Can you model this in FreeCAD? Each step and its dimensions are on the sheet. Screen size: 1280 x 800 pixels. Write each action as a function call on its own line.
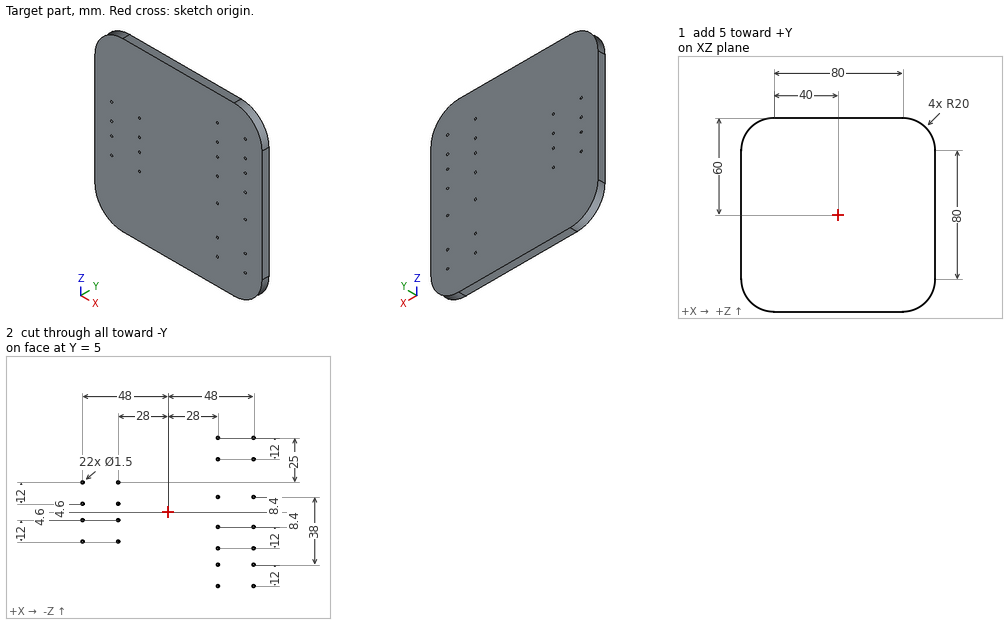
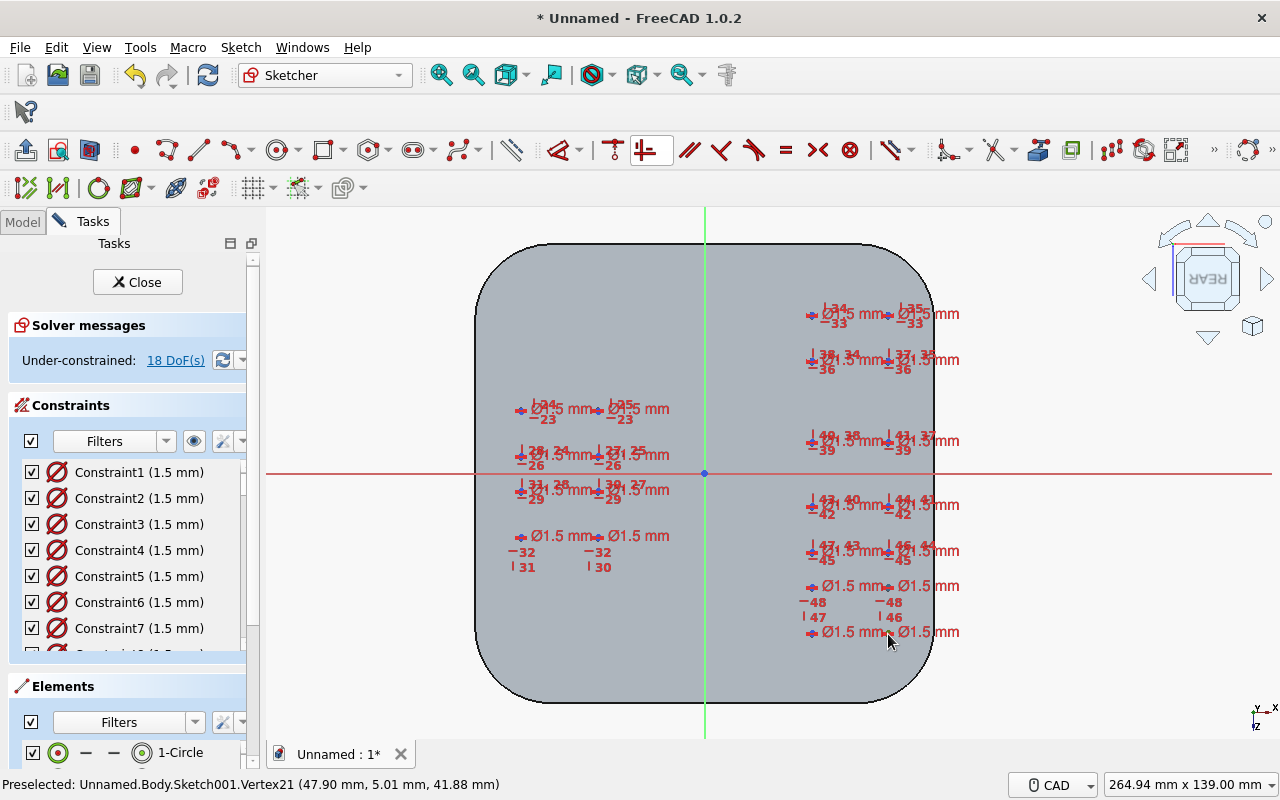
click(668, 150)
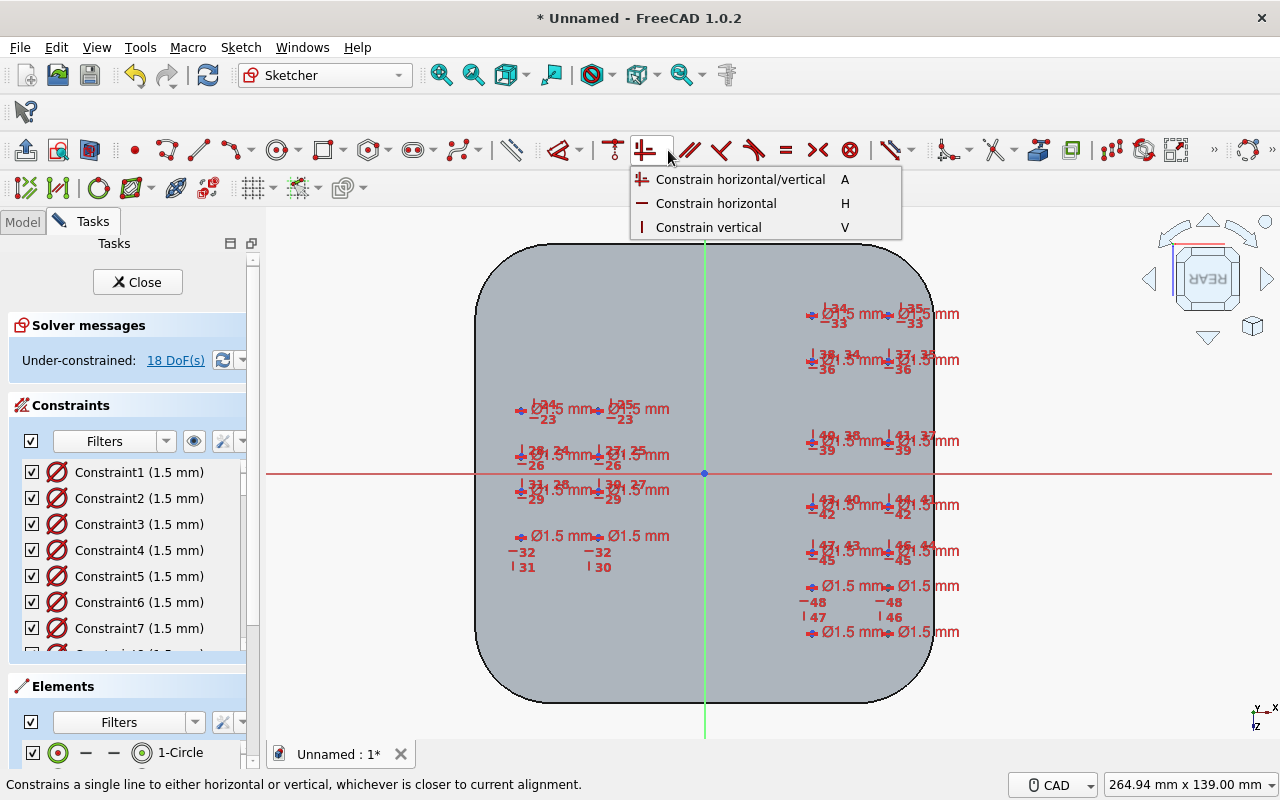
click(766, 227)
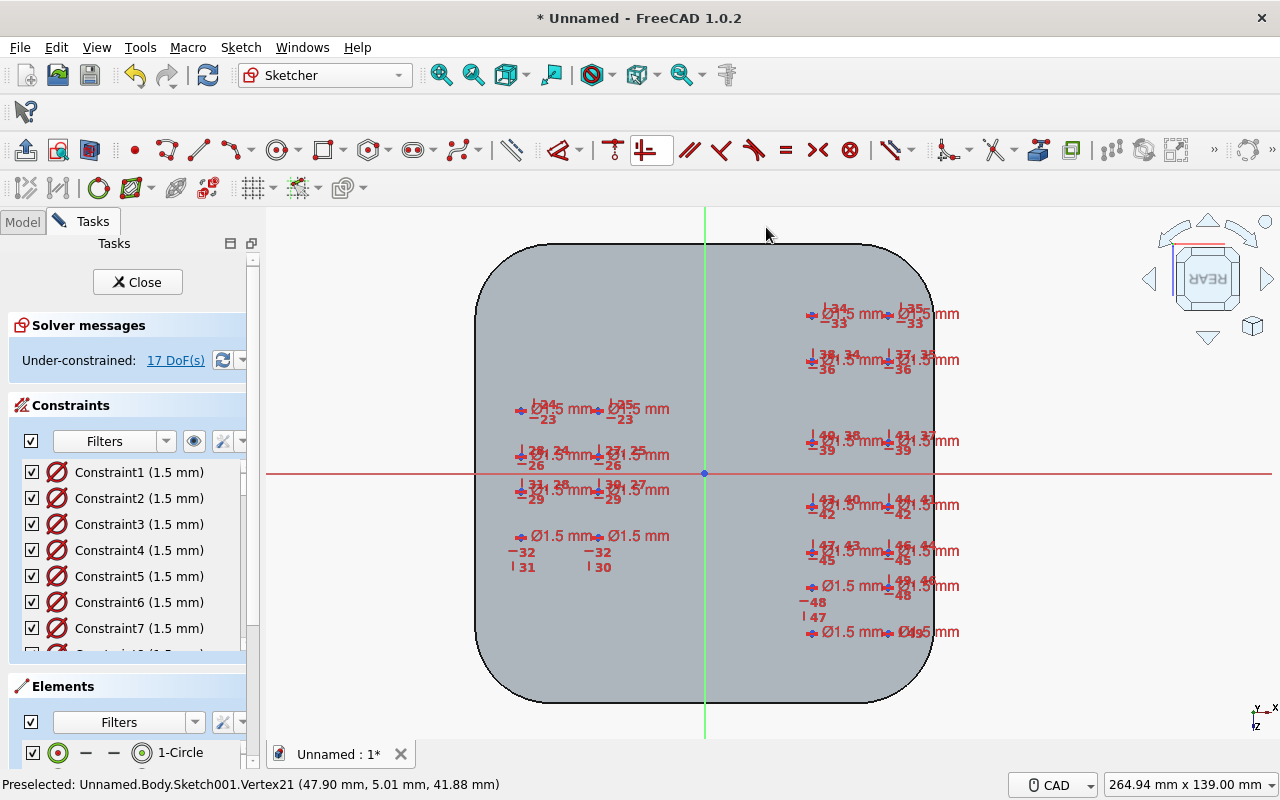
click(812, 588)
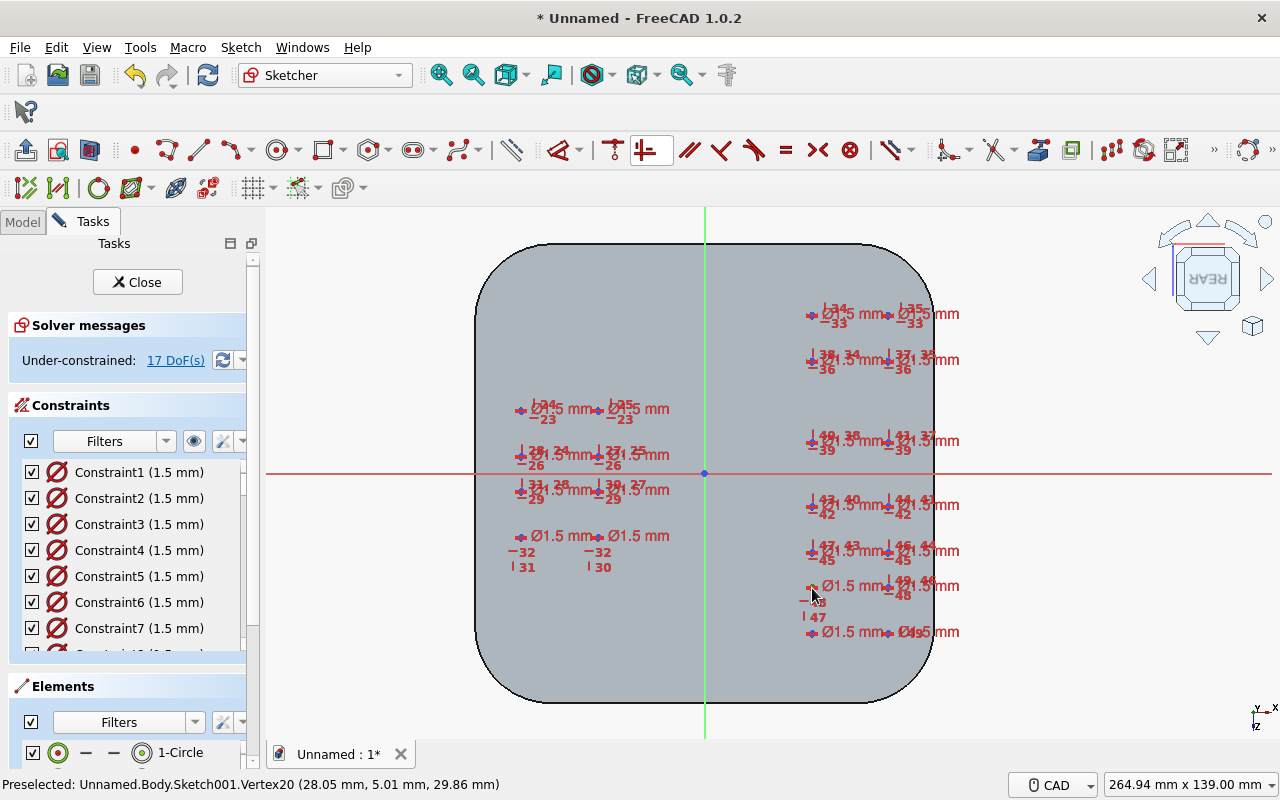
click(812, 634)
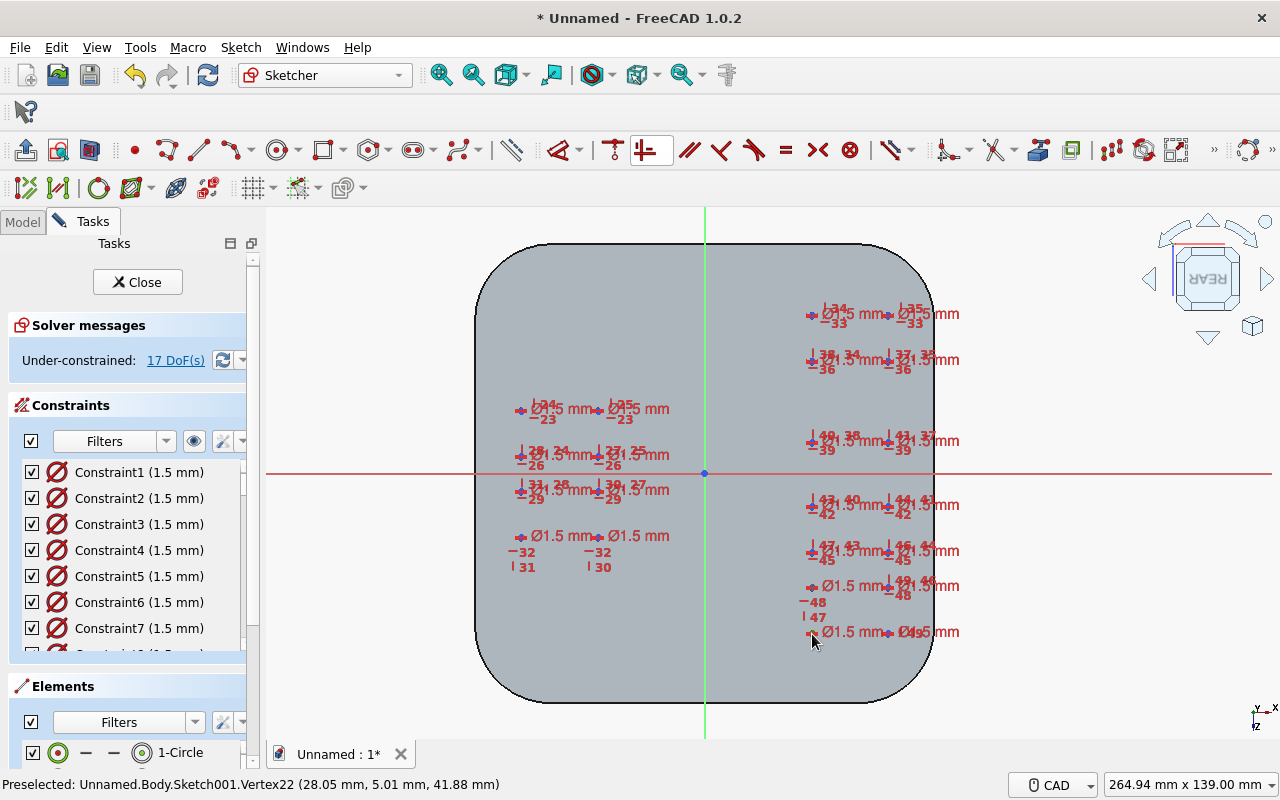
click(668, 150)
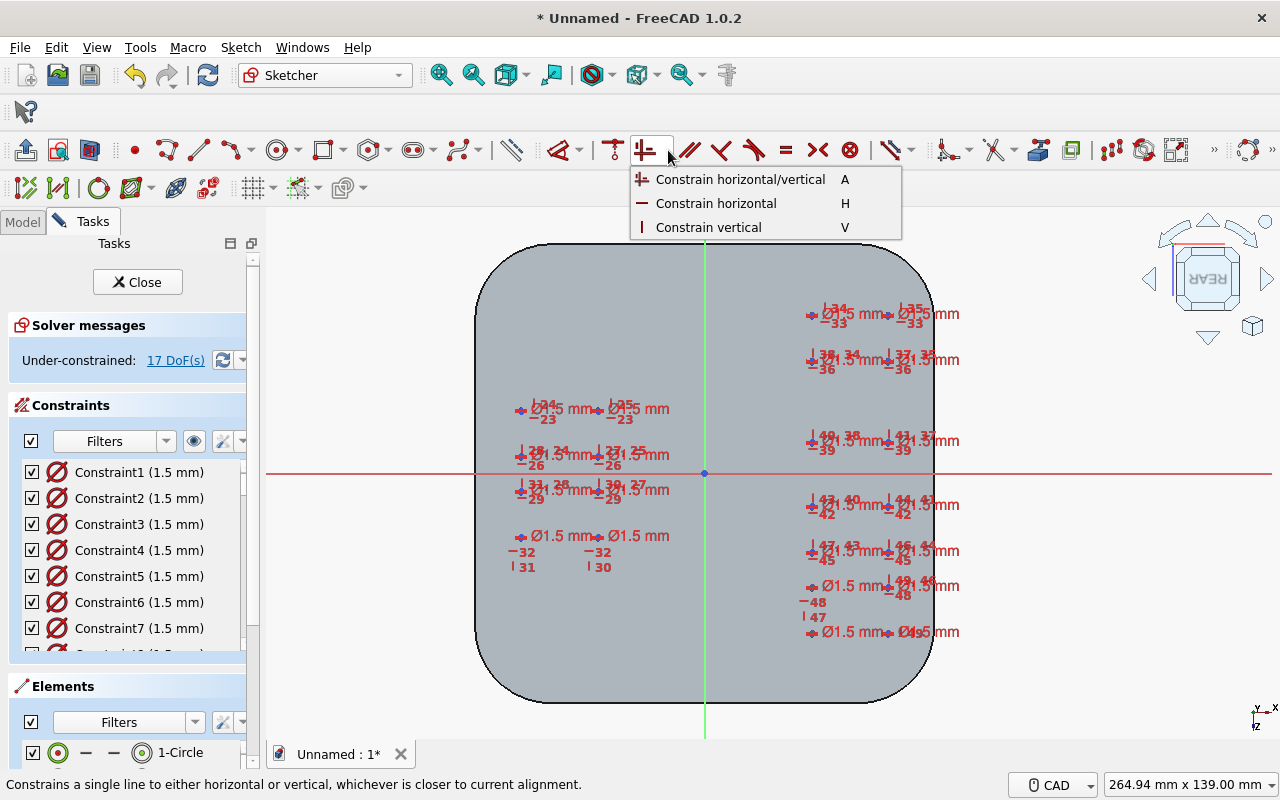
click(766, 227)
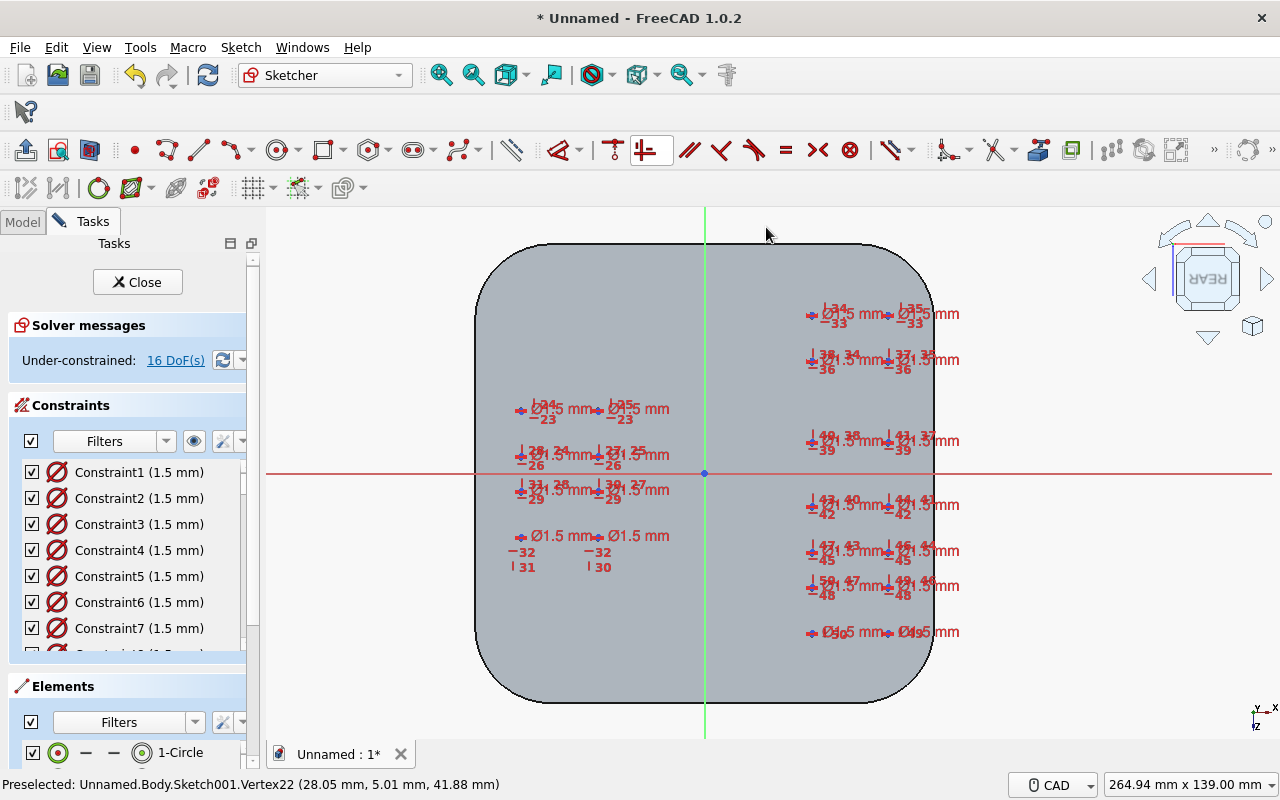
click(888, 634)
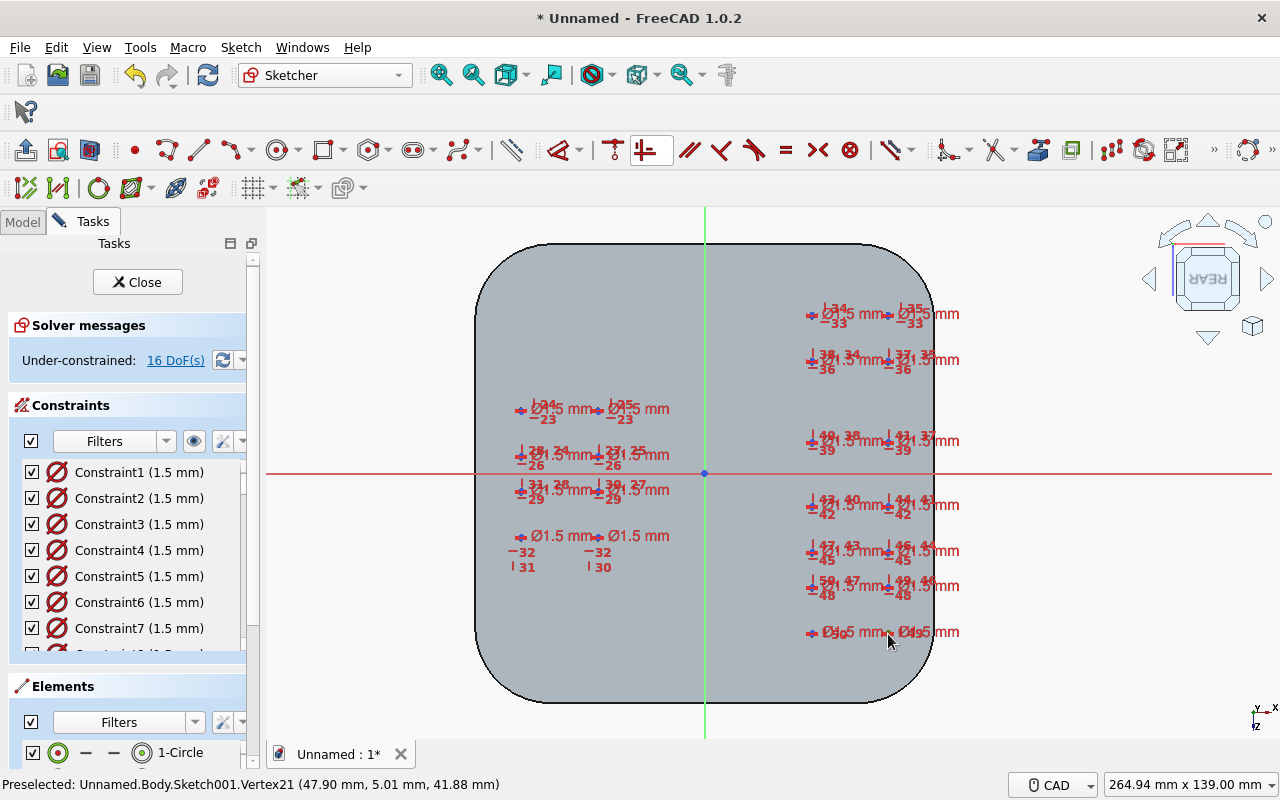
click(812, 634)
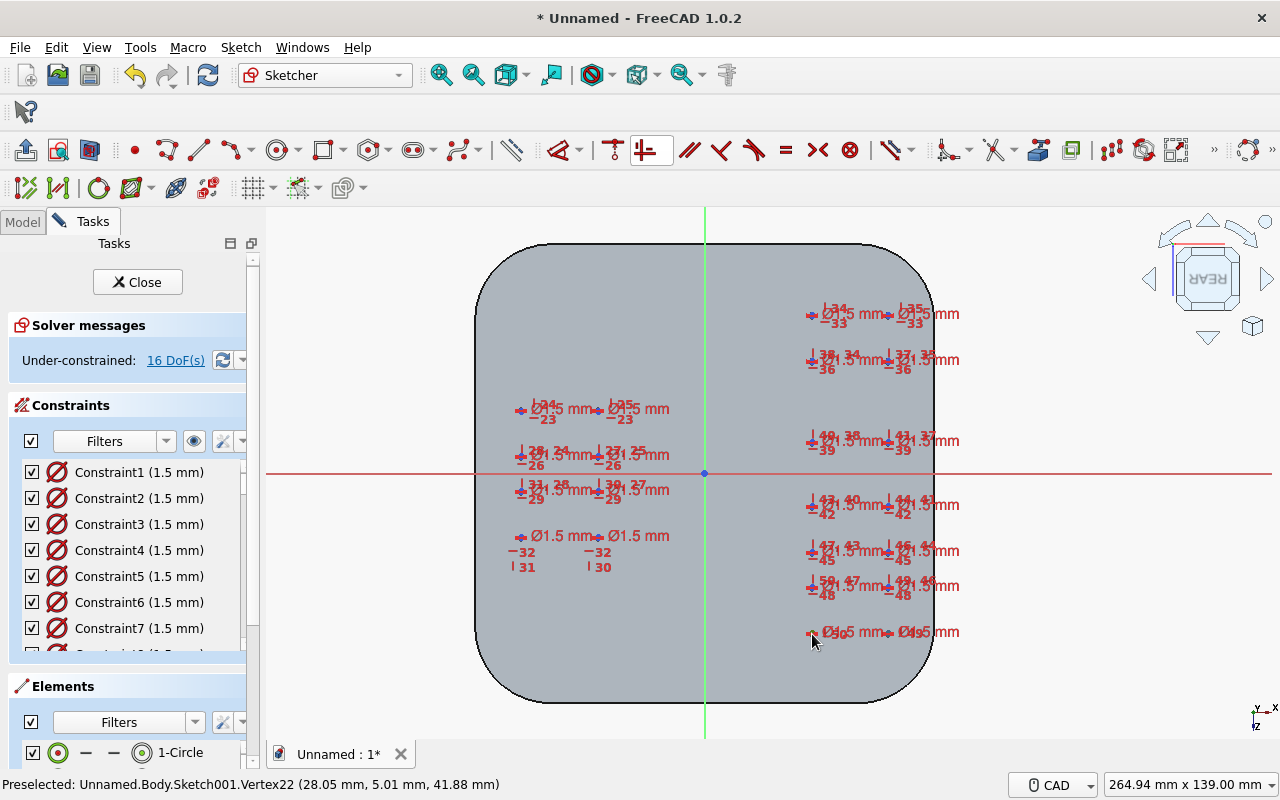
click(668, 150)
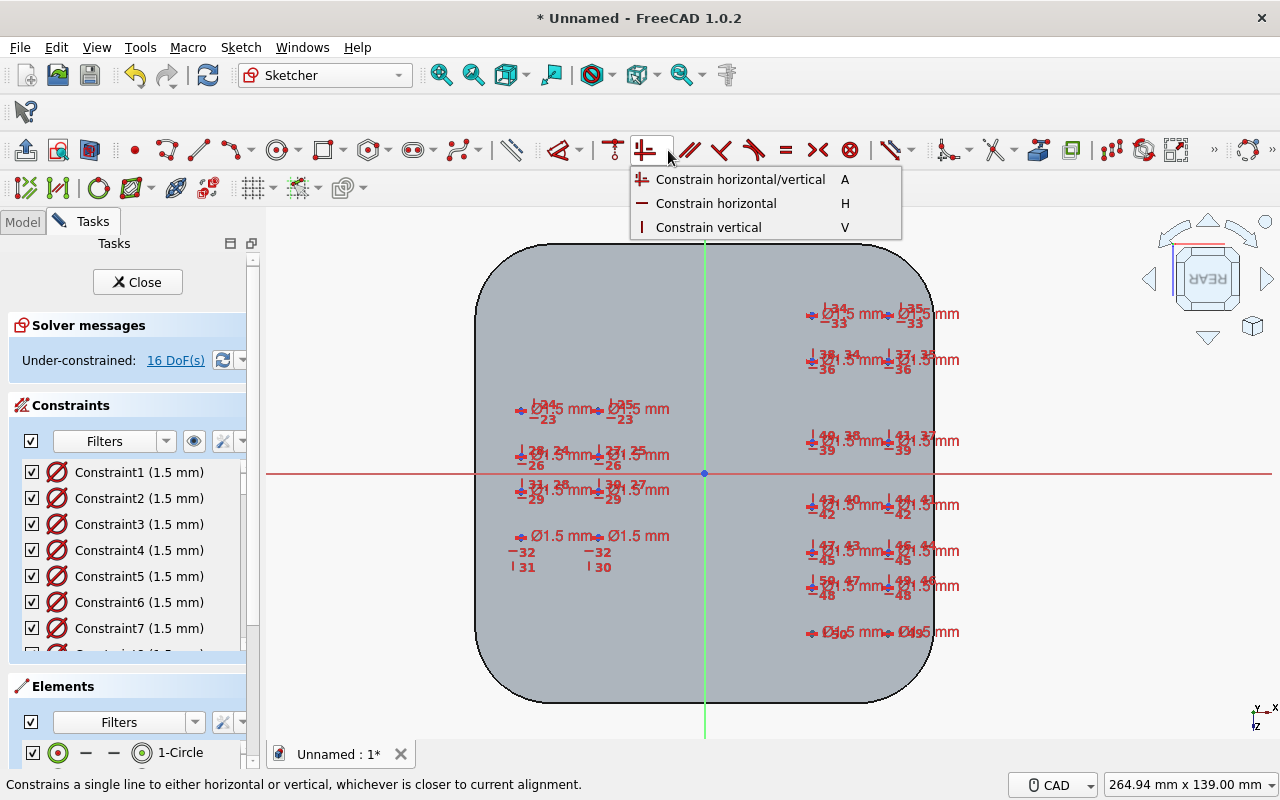
click(766, 203)